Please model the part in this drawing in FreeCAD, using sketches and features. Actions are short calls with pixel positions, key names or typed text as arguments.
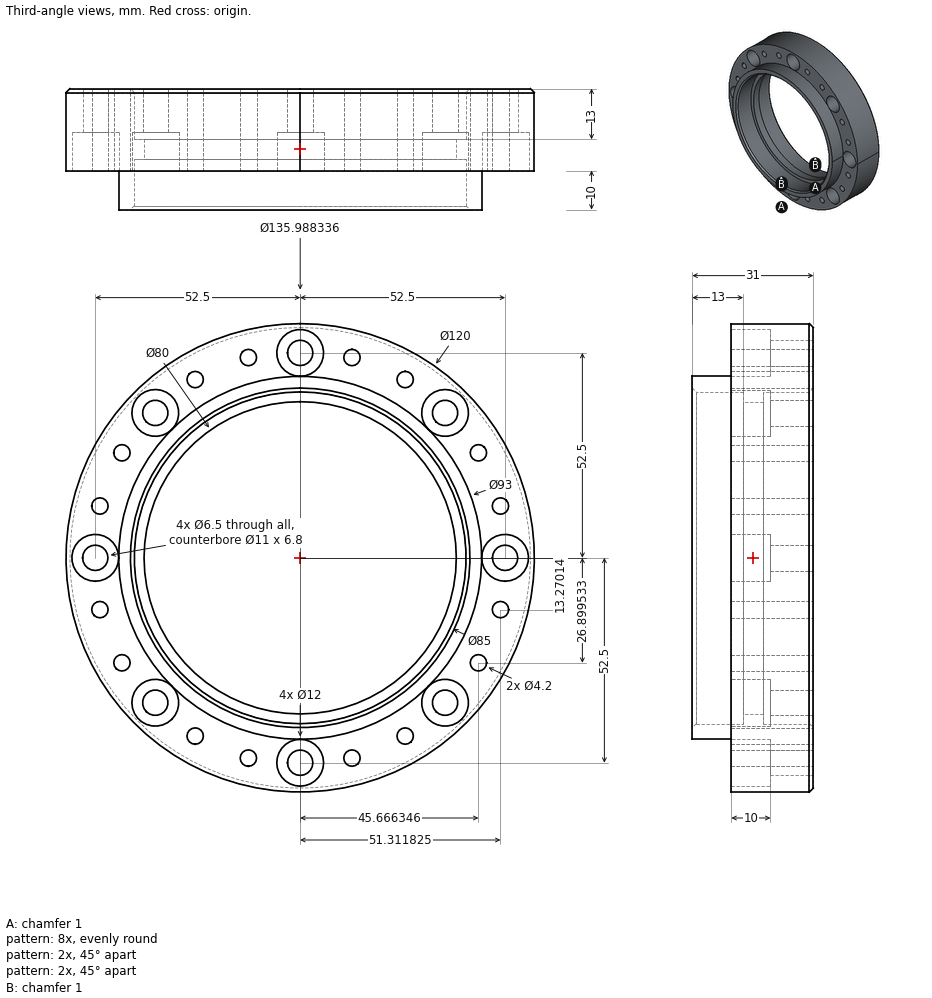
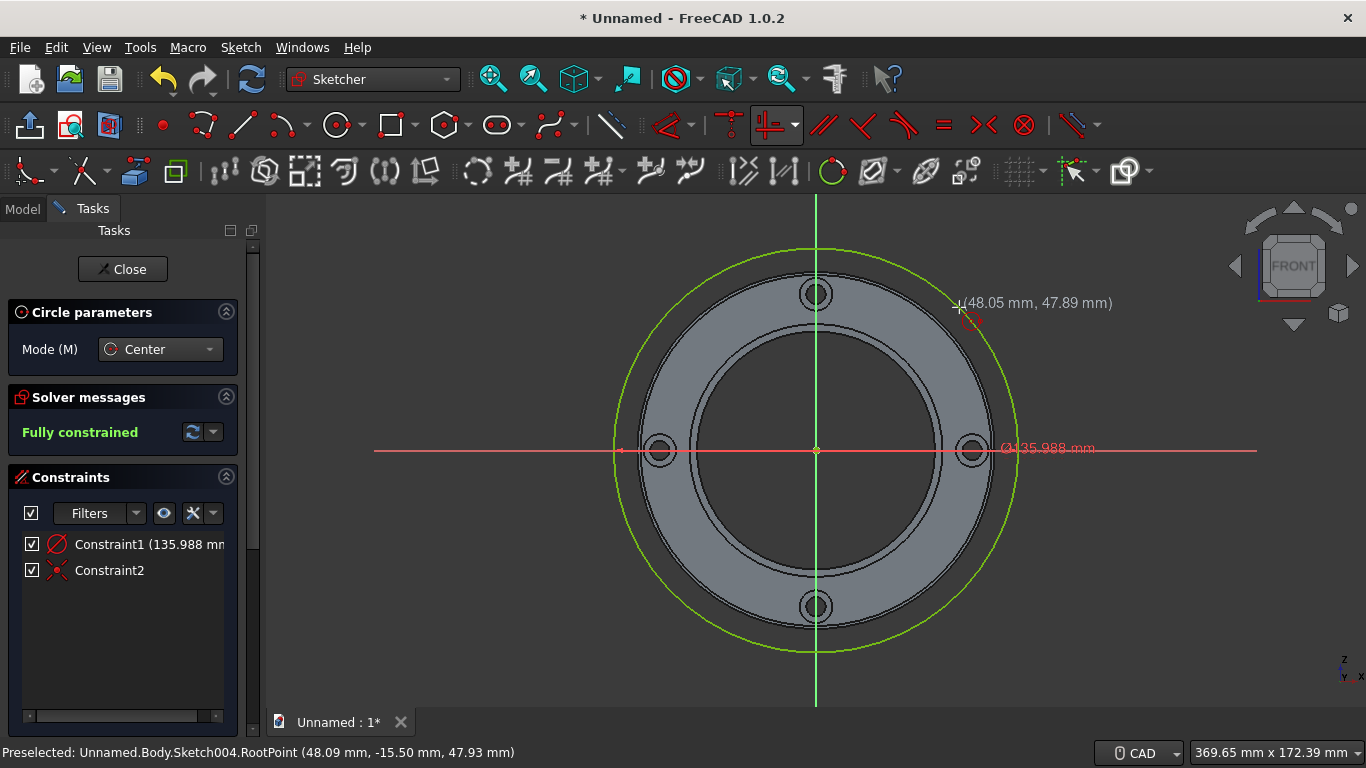
click(816, 451)
move(914, 353)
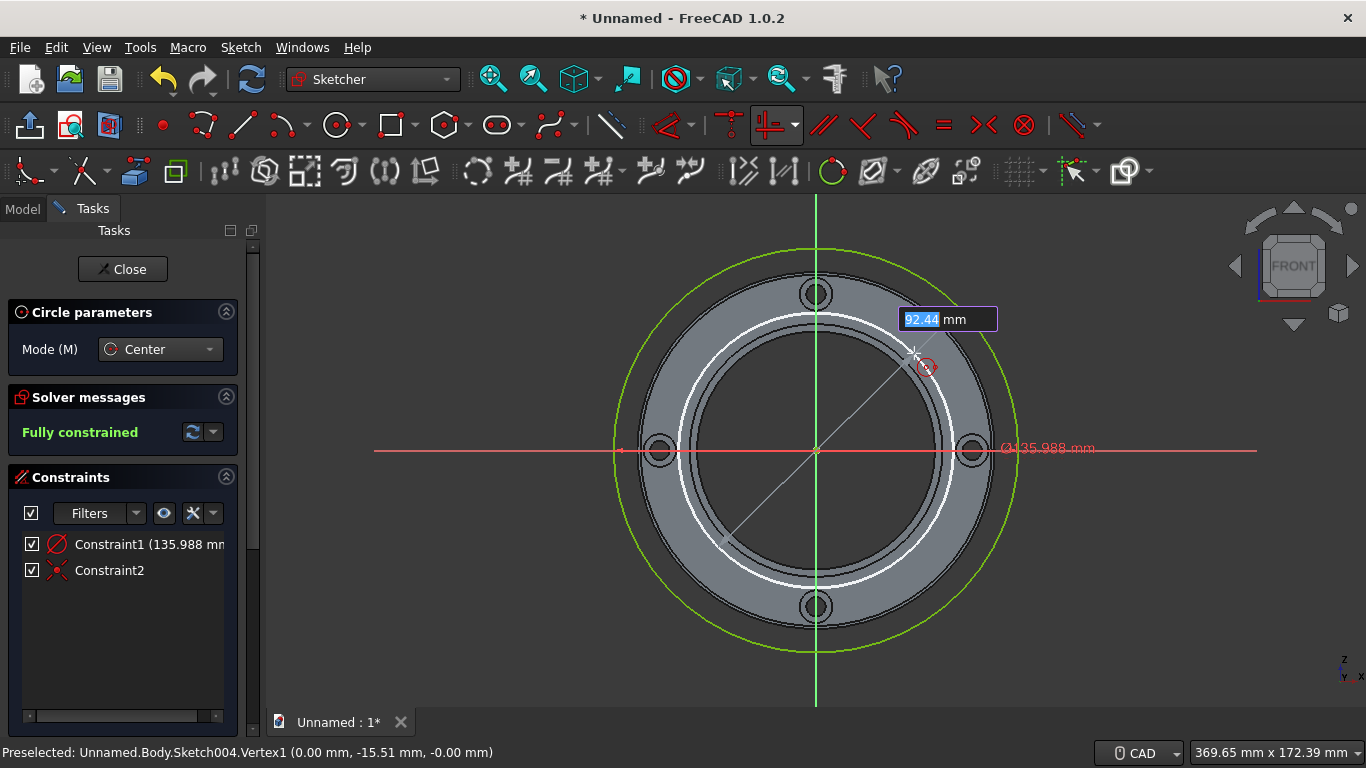
text(93)
key(Return)
key(Escape)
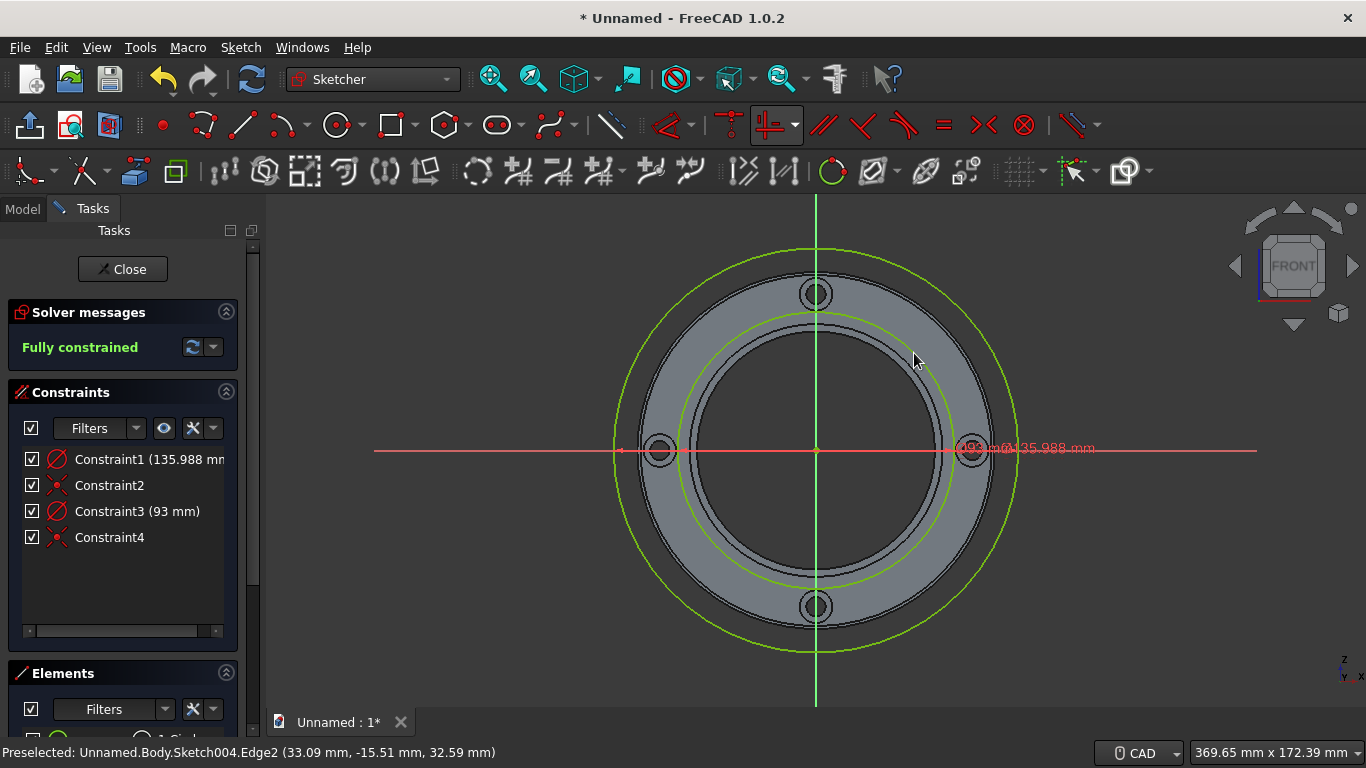
click(123, 269)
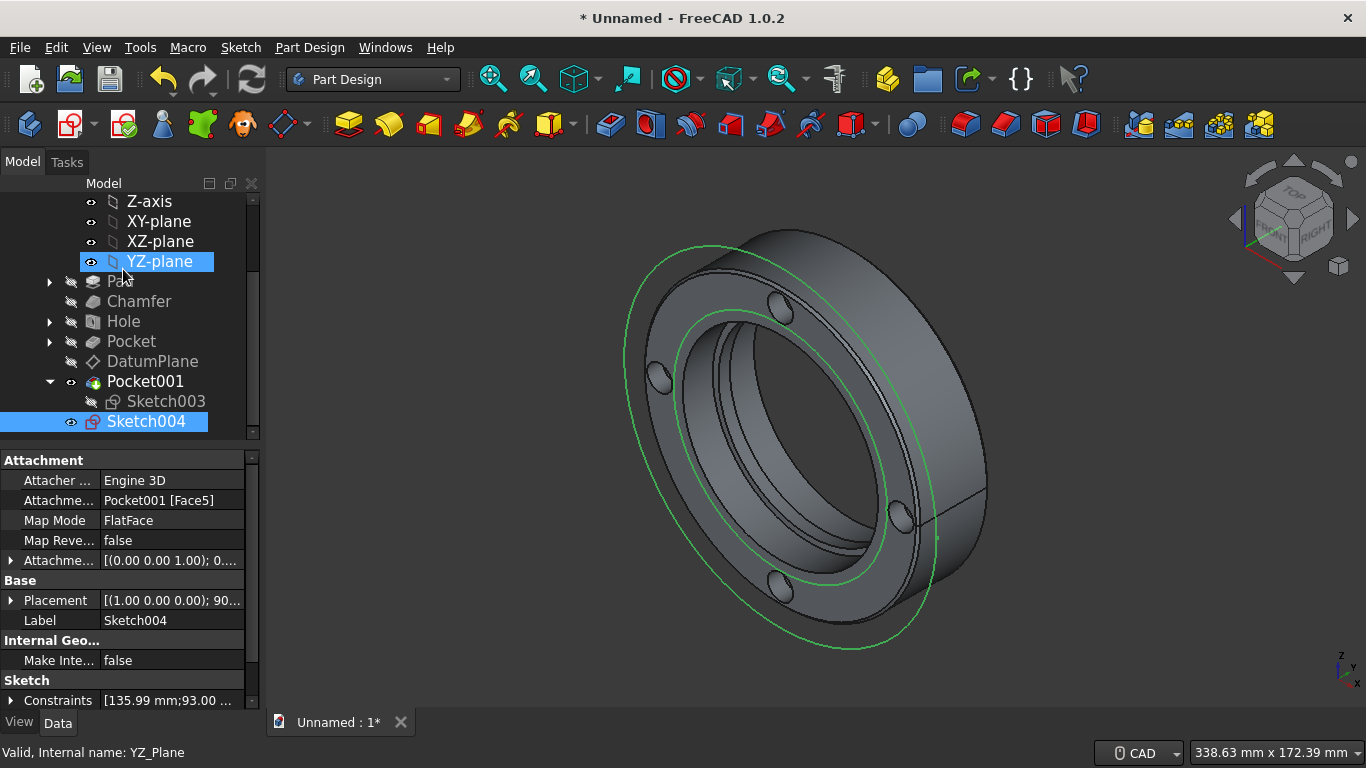
click(612, 124)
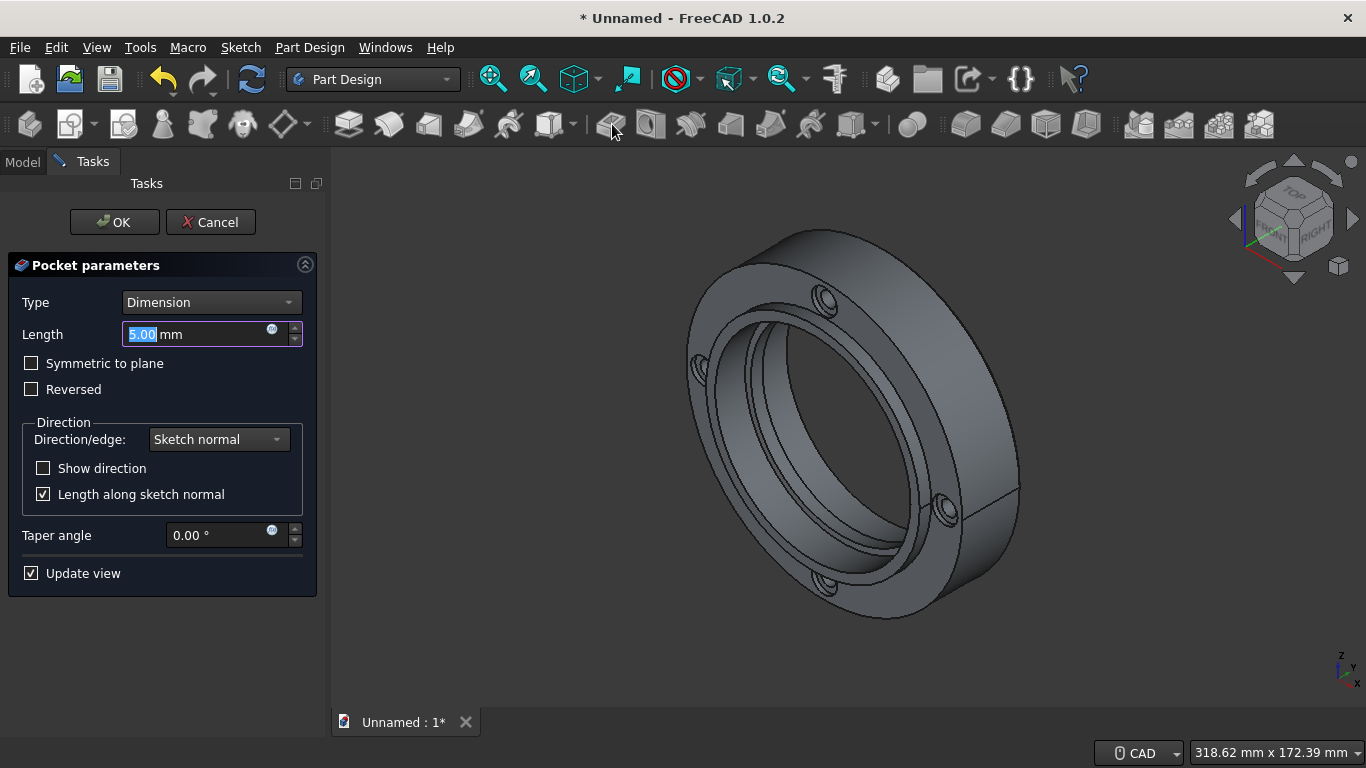
text(10)
key(Tab)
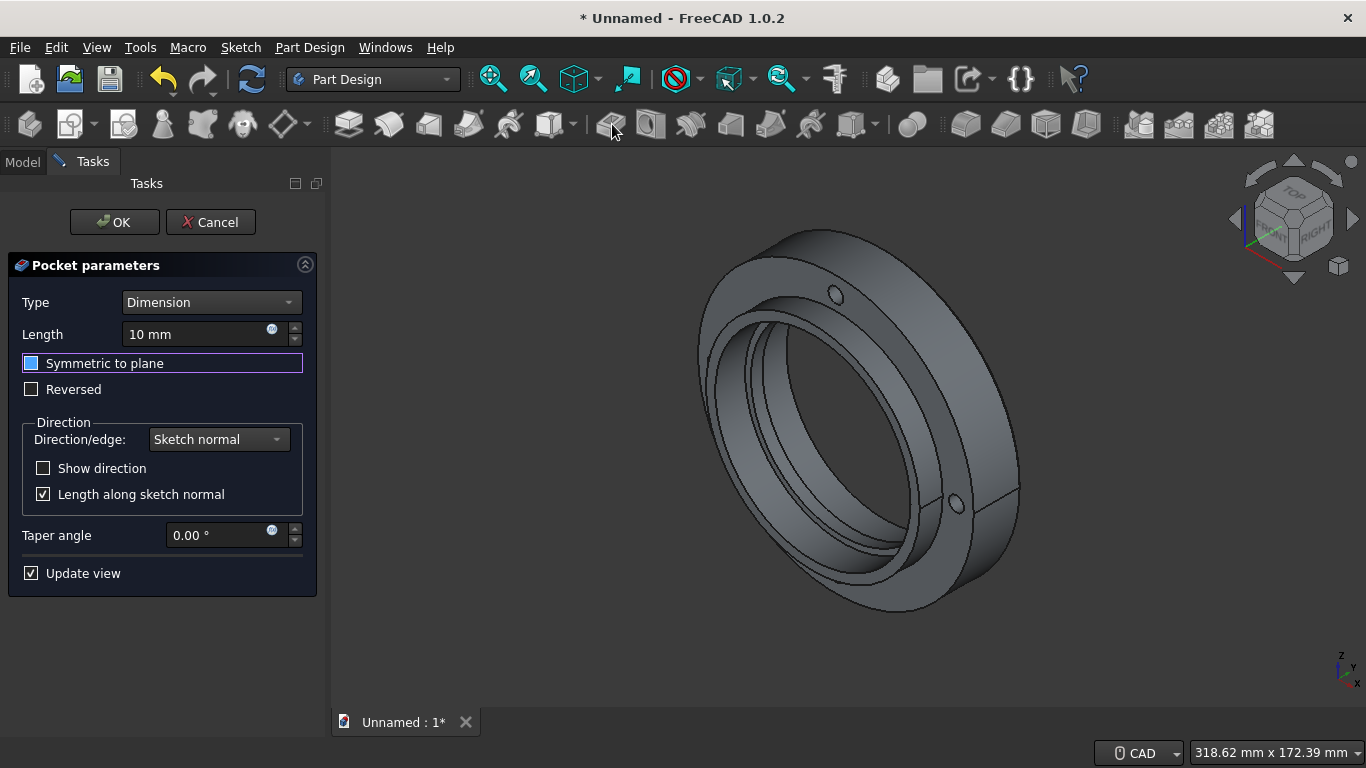
click(115, 222)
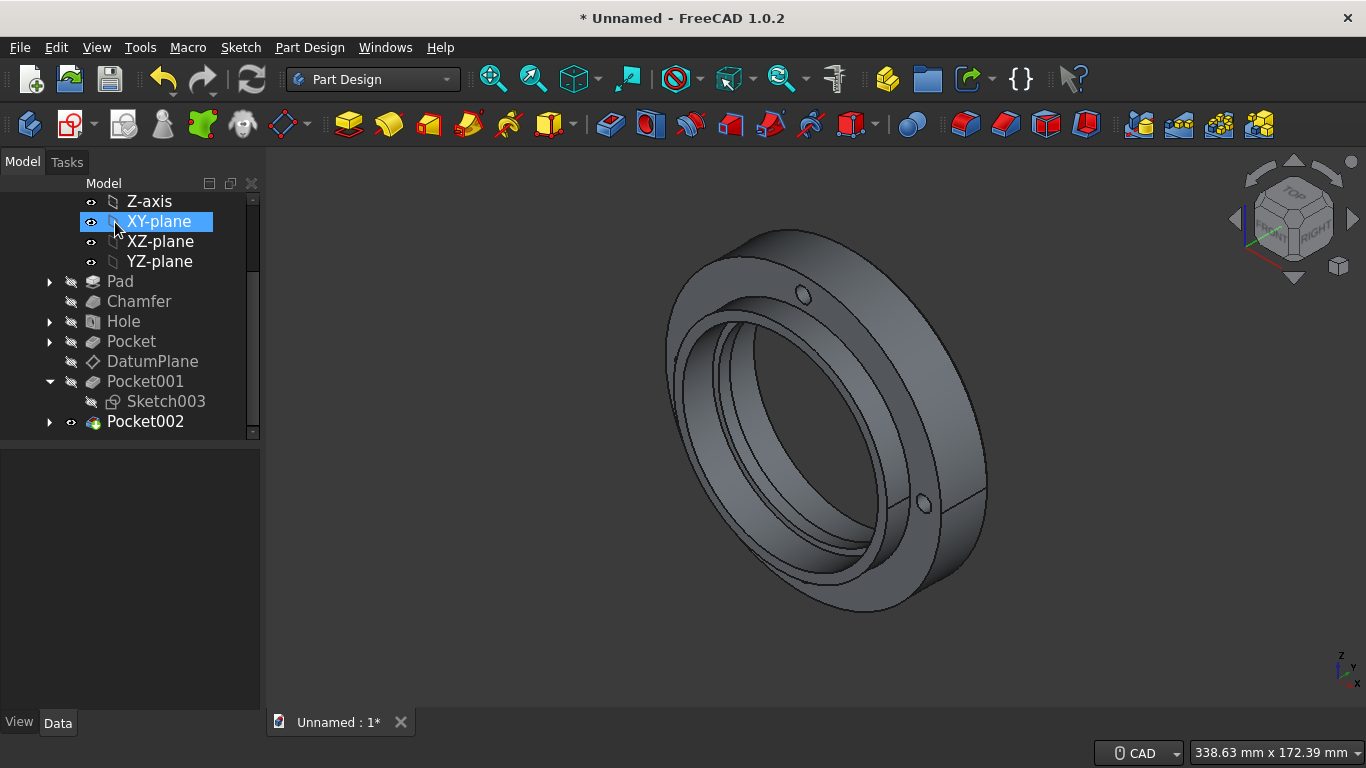
click(685, 320)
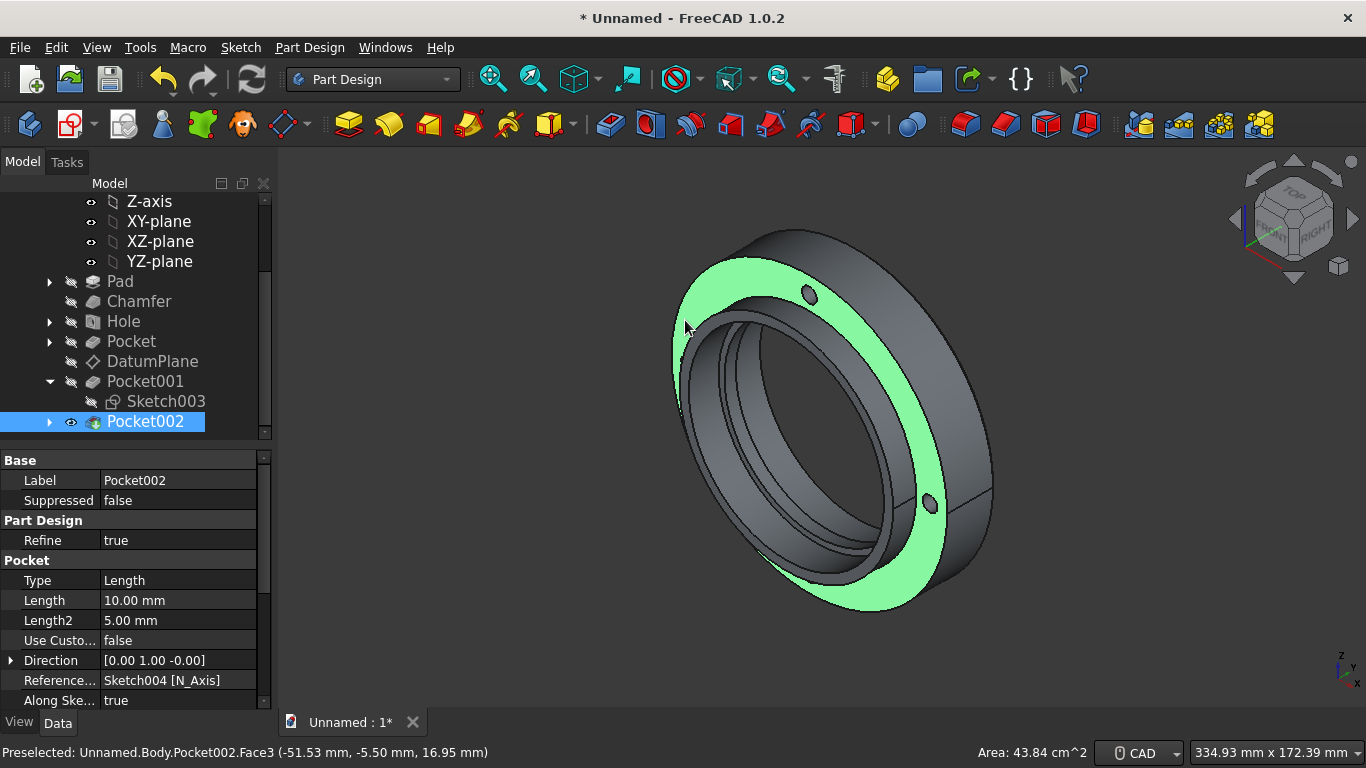
click(70, 124)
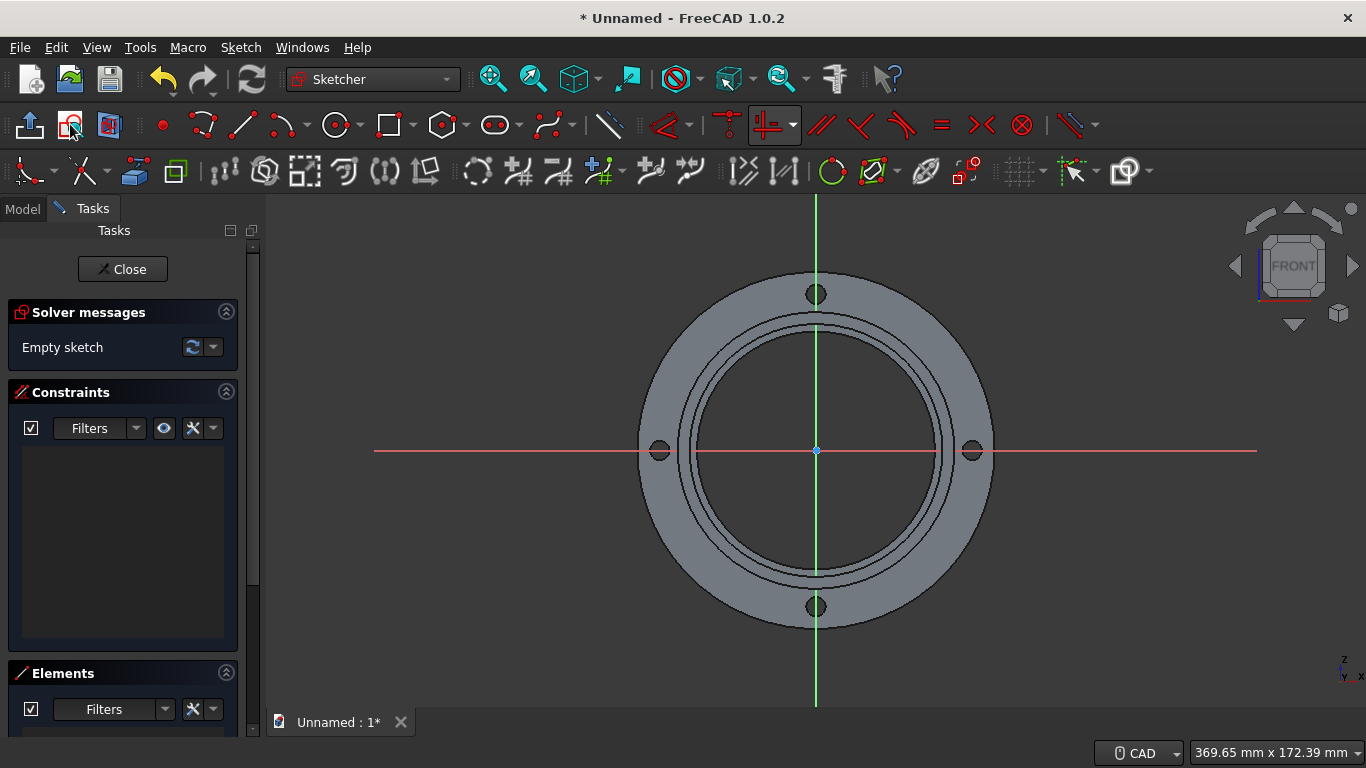
scroll(1002, 522, up, 9)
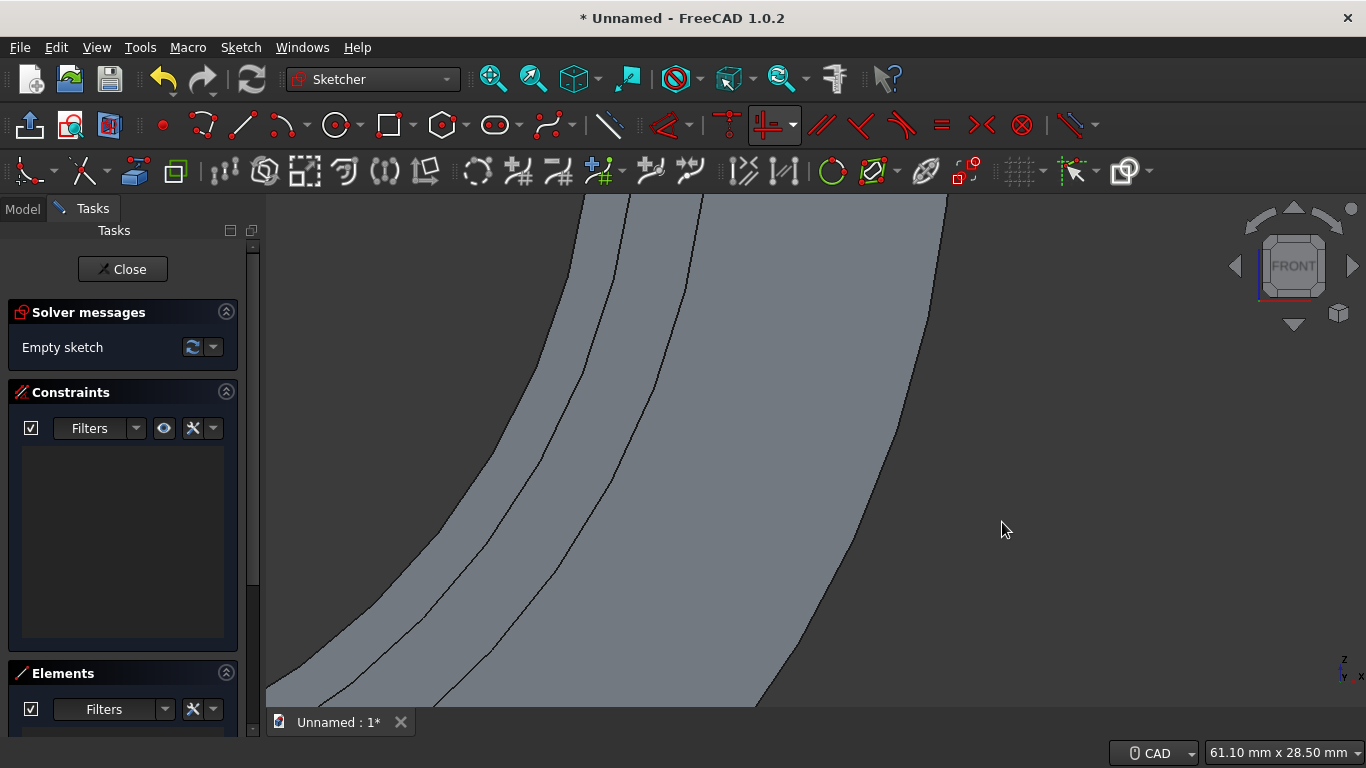
click(336, 126)